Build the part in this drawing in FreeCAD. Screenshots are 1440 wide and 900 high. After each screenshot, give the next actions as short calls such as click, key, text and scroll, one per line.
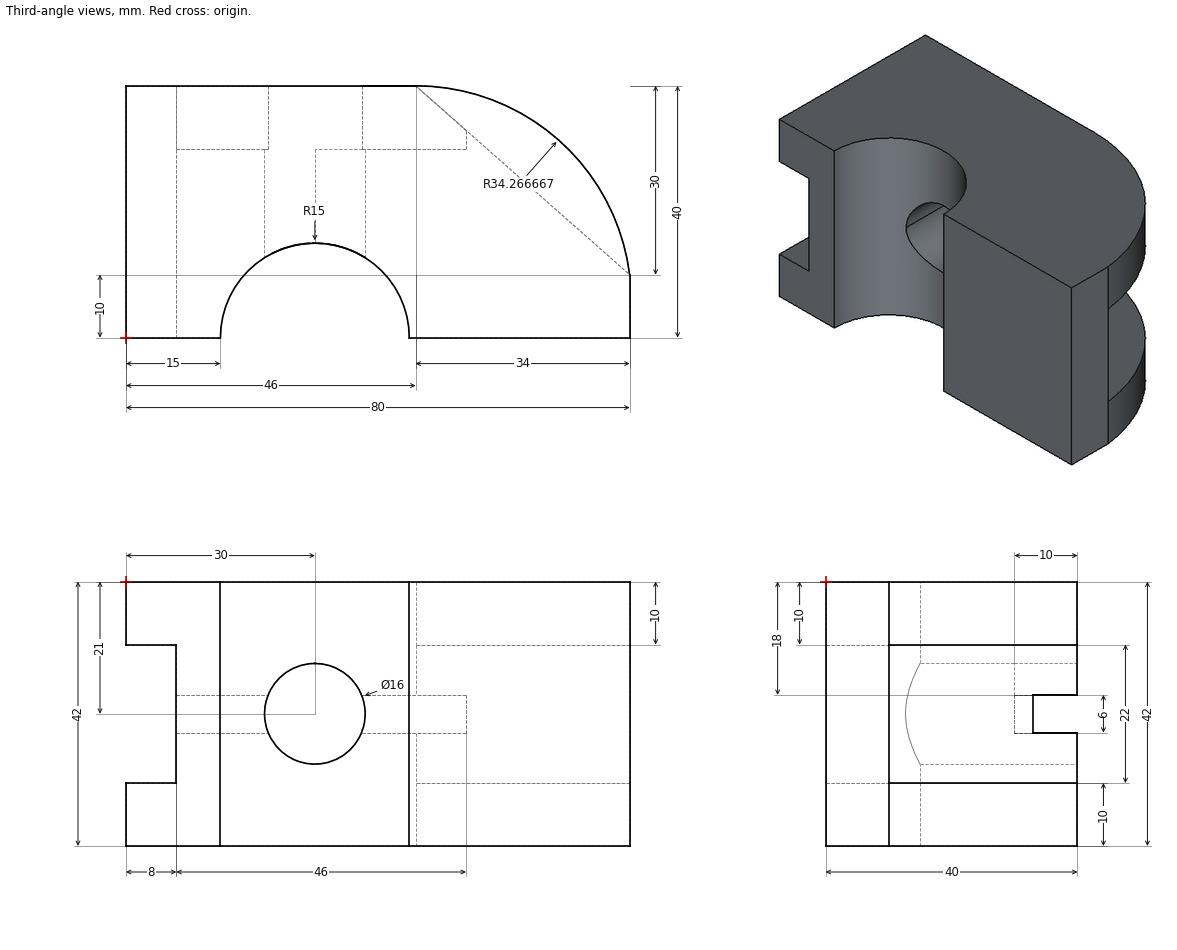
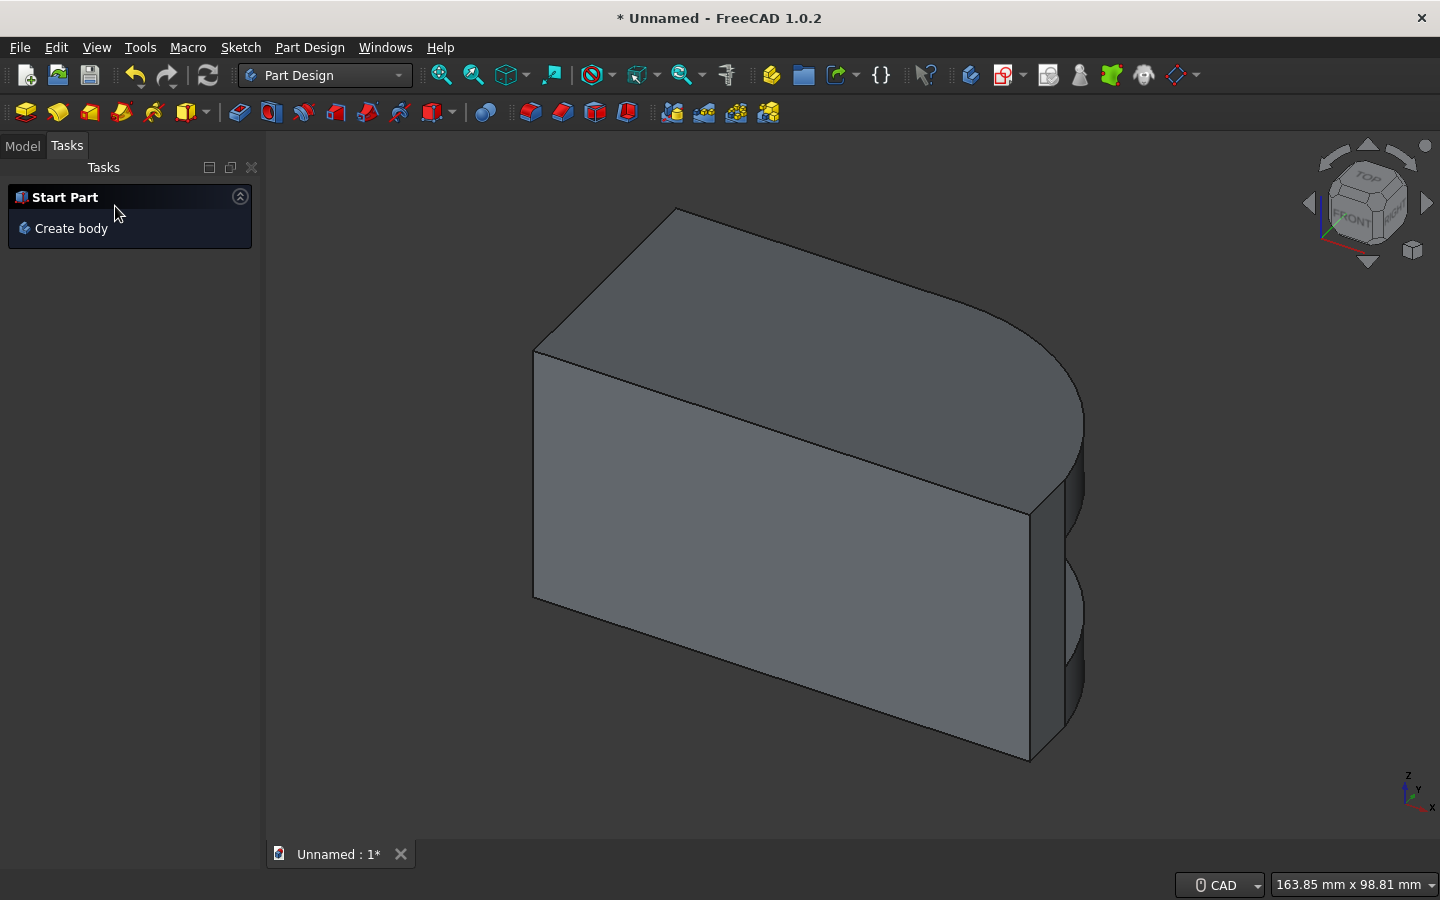
click(1004, 76)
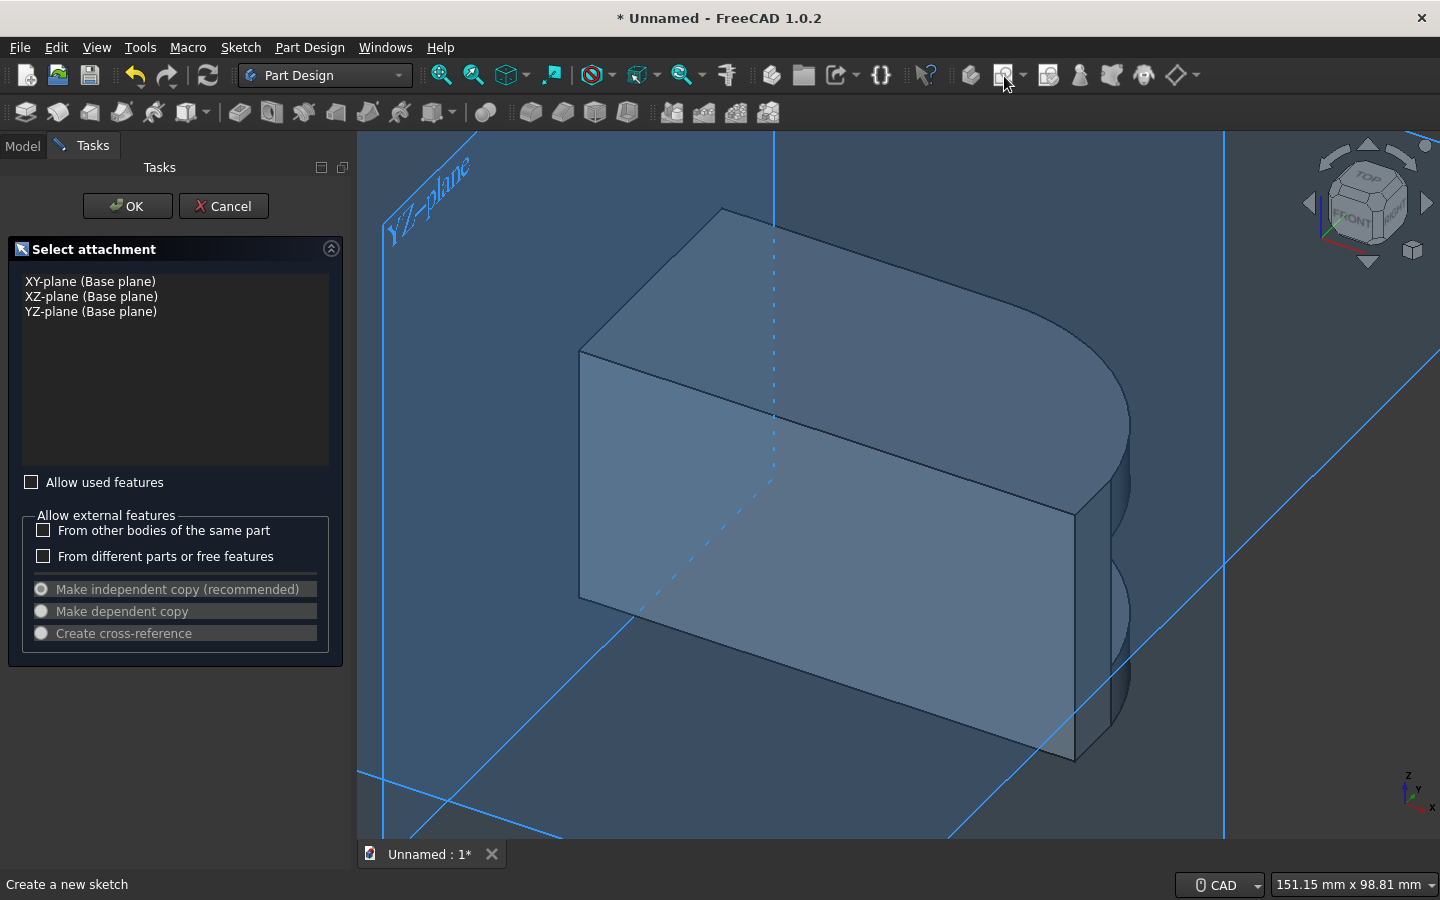
click(82, 282)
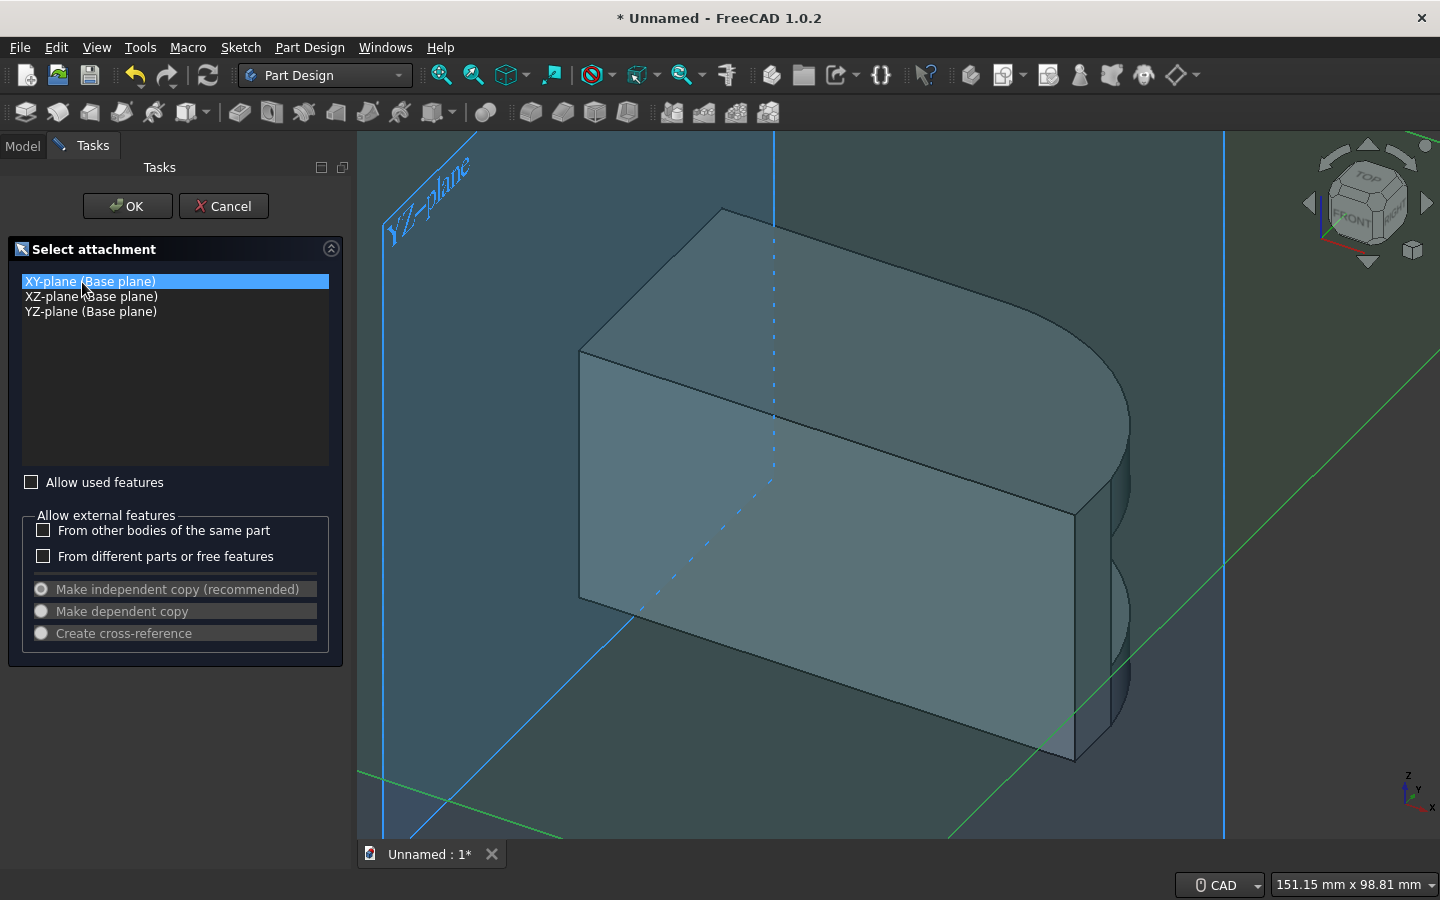
click(128, 206)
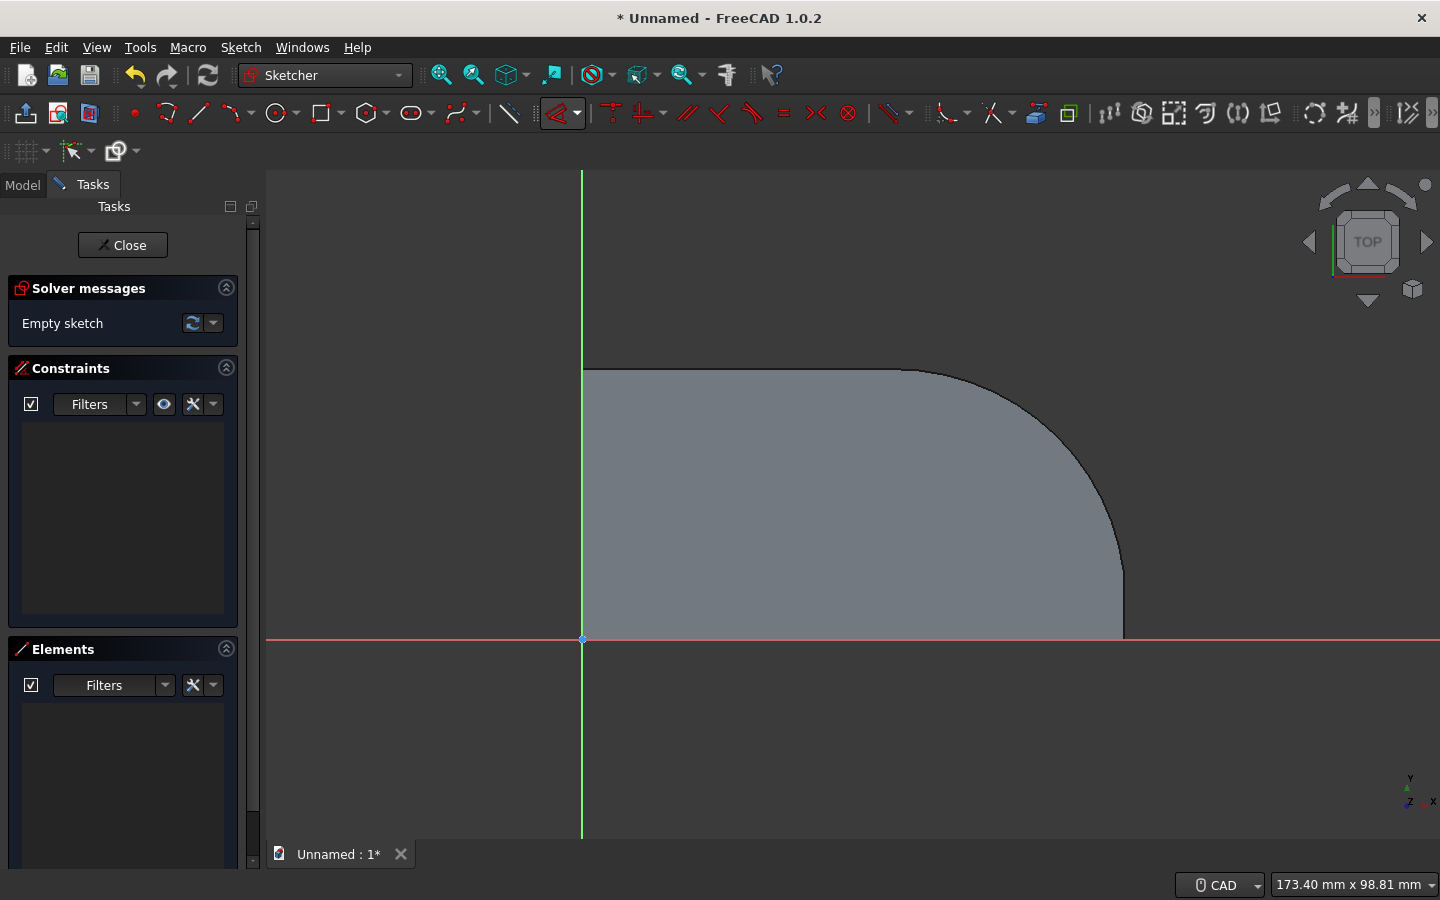
scroll(694, 658, up, 4)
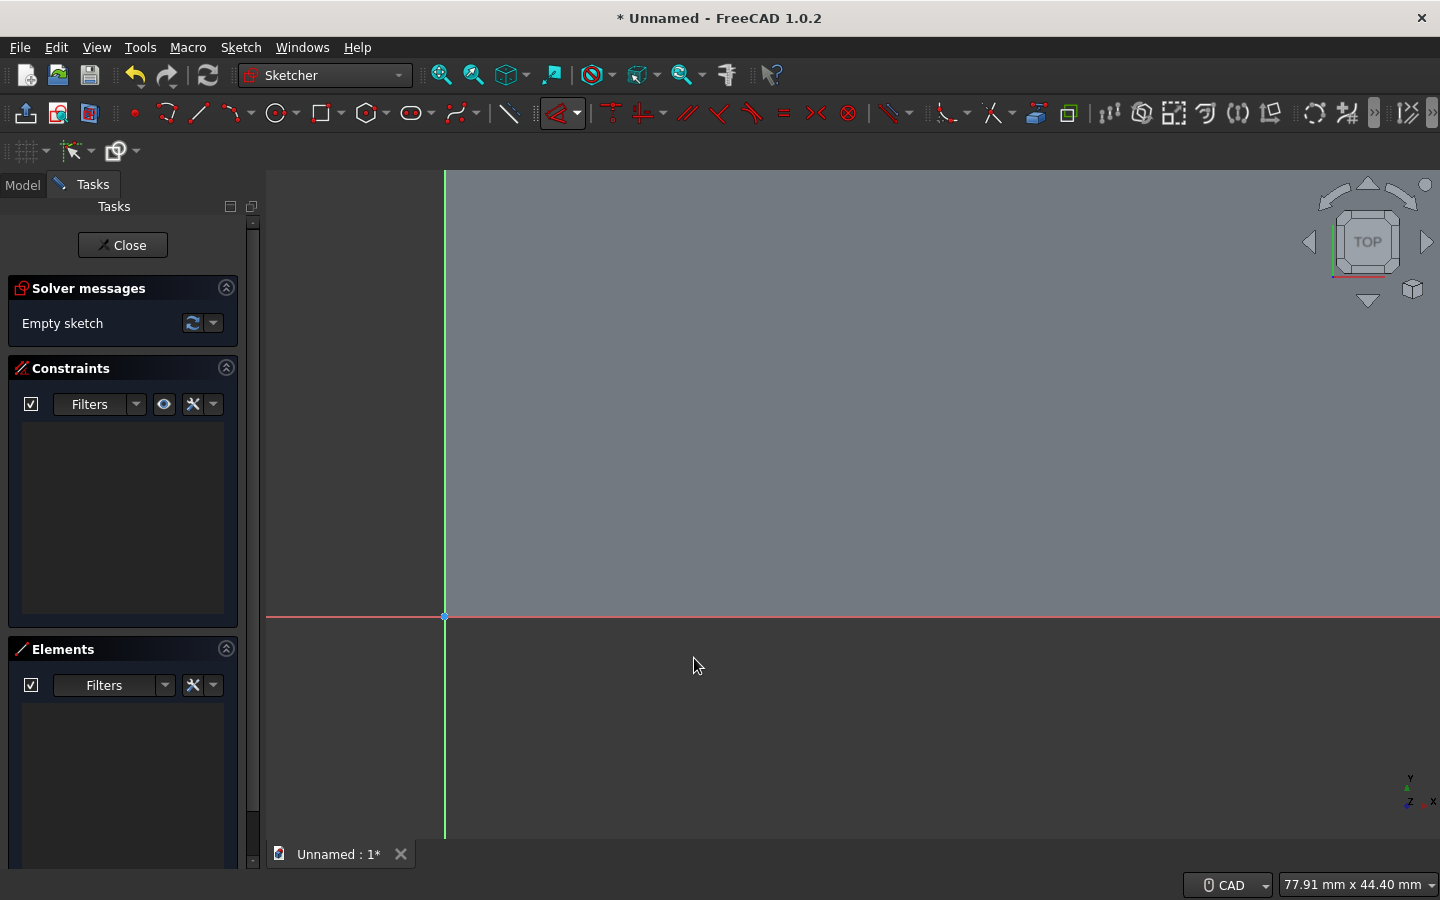
click(200, 114)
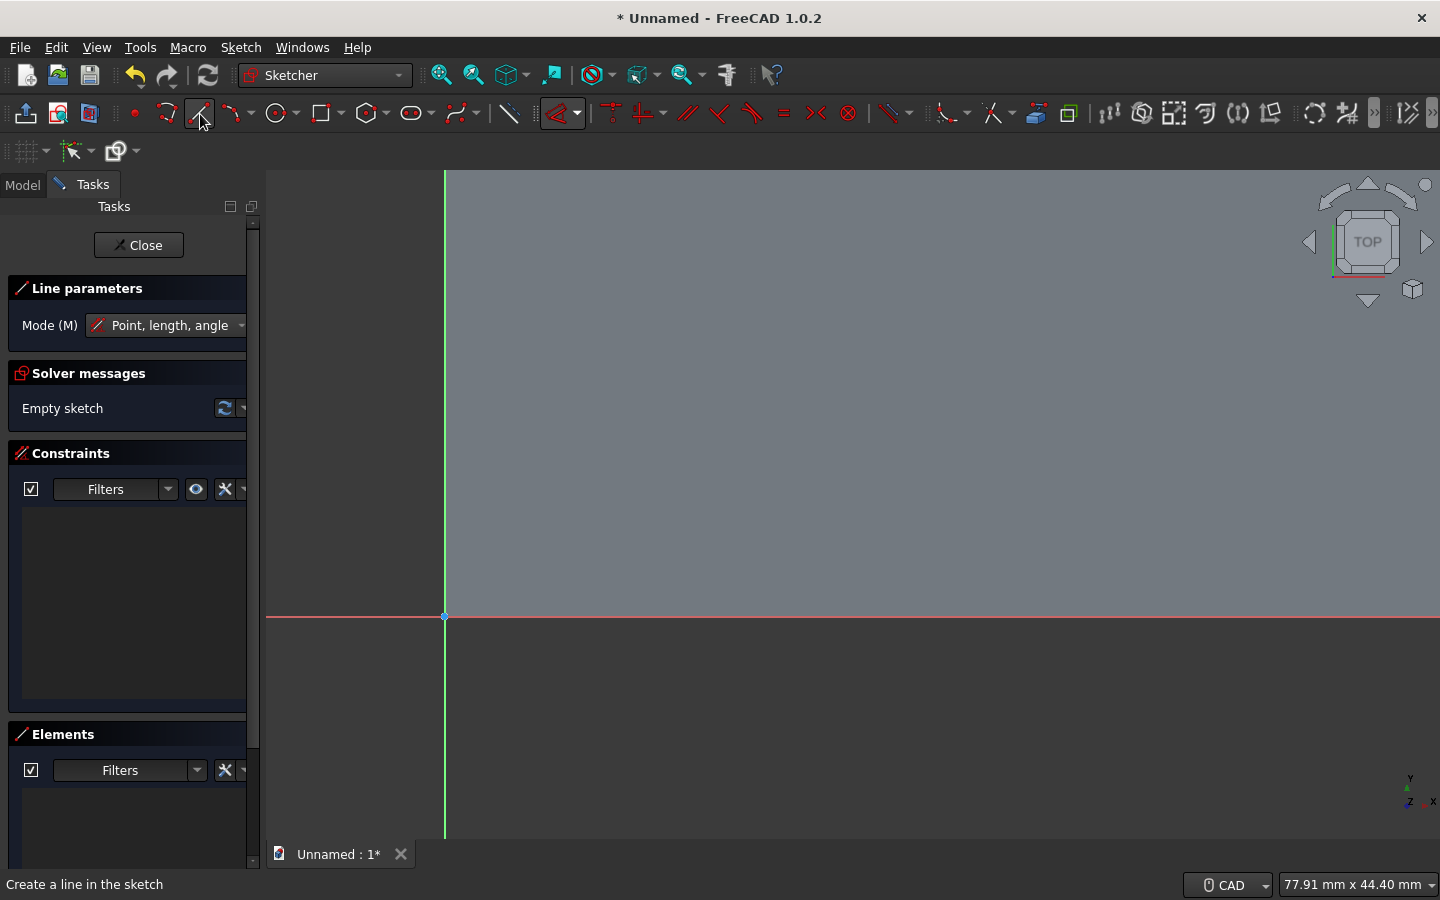
click(671, 617)
click(1123, 608)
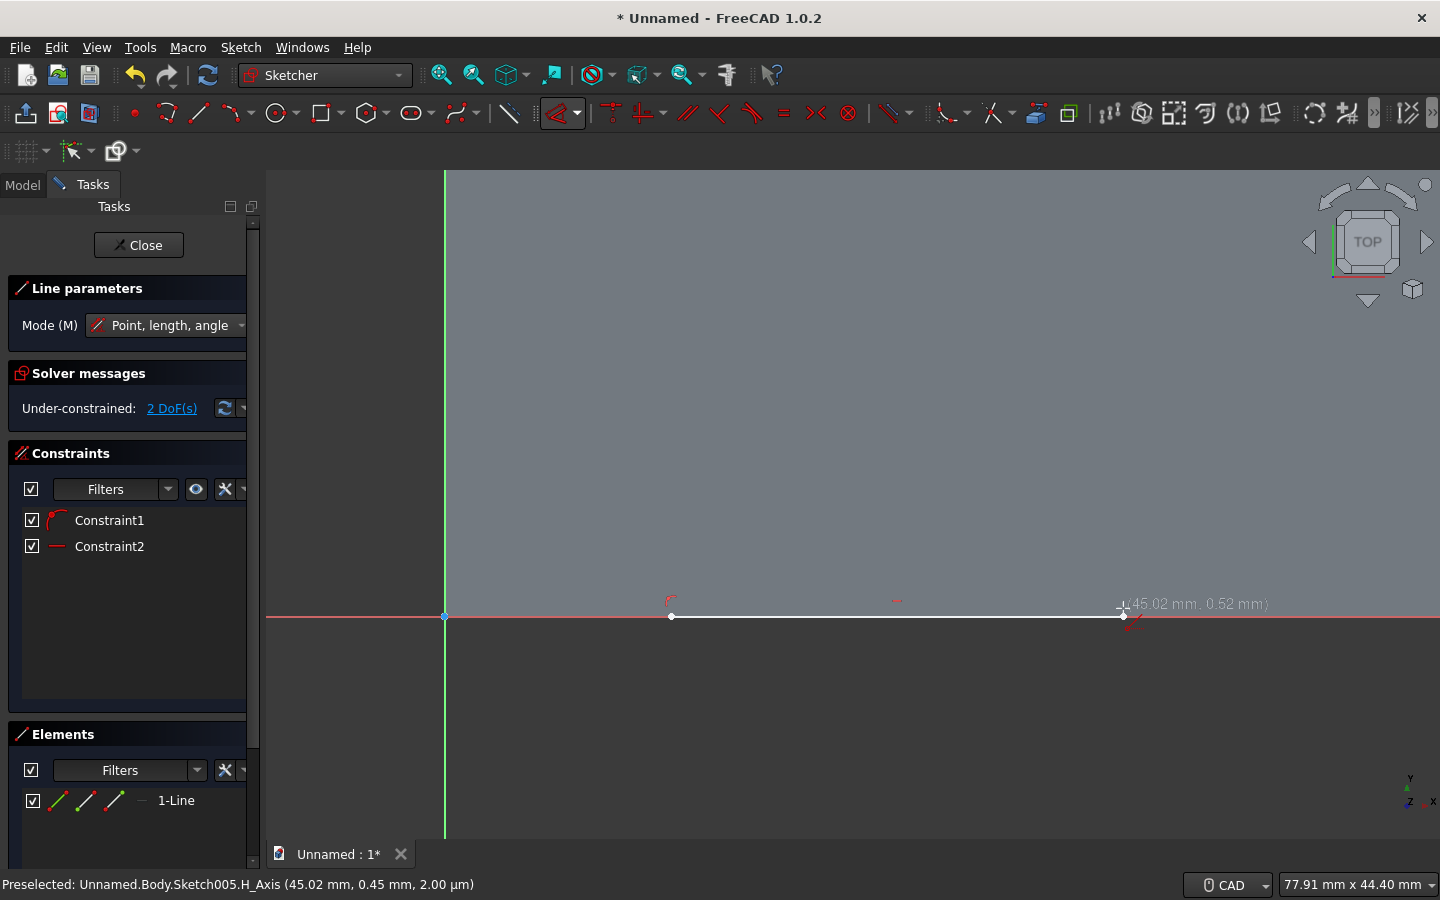
click(232, 114)